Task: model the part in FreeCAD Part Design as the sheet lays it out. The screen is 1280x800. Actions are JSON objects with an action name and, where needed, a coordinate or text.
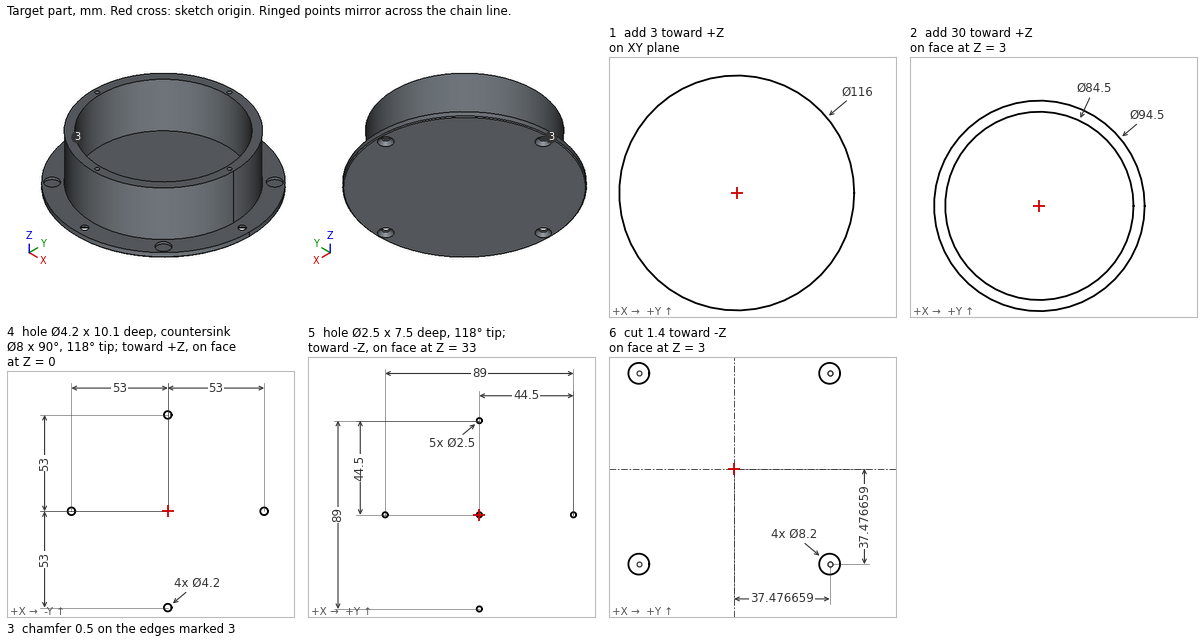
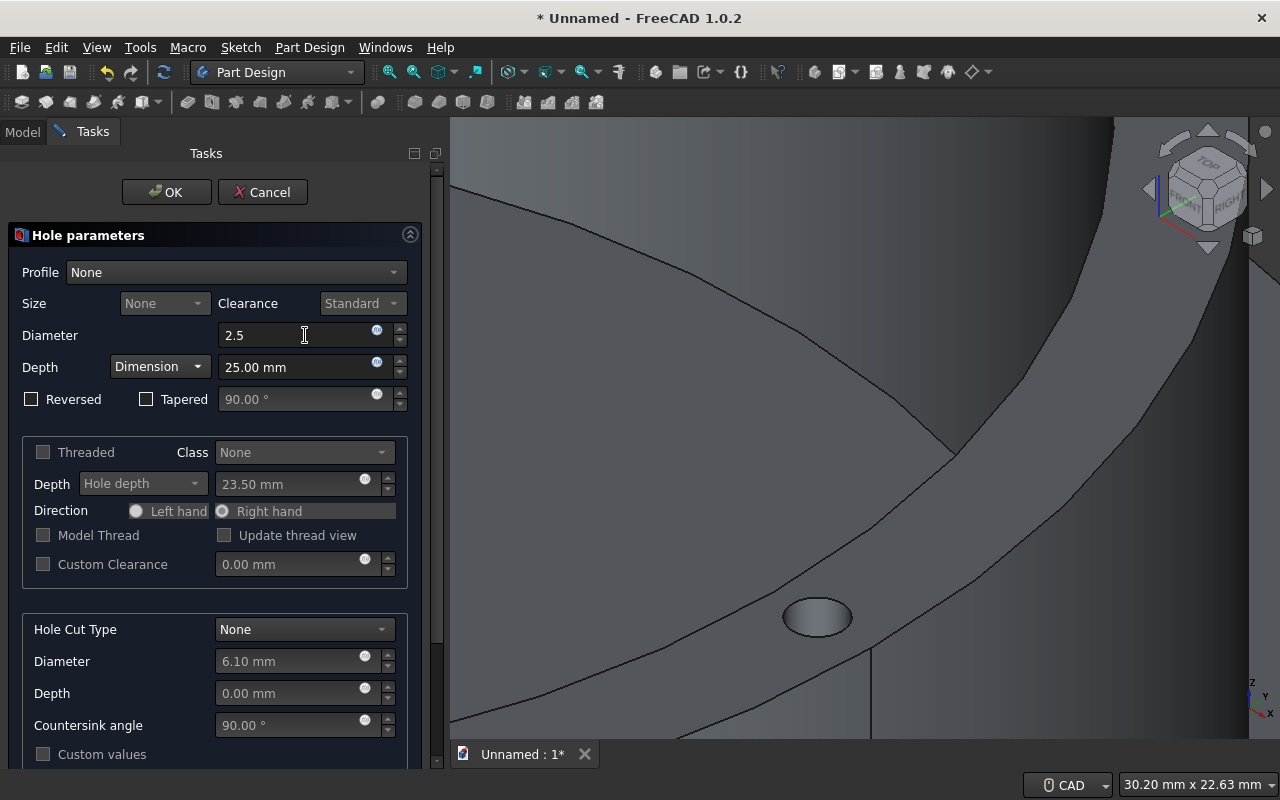
{"action": "triple_click", "coordinate": [305, 367]}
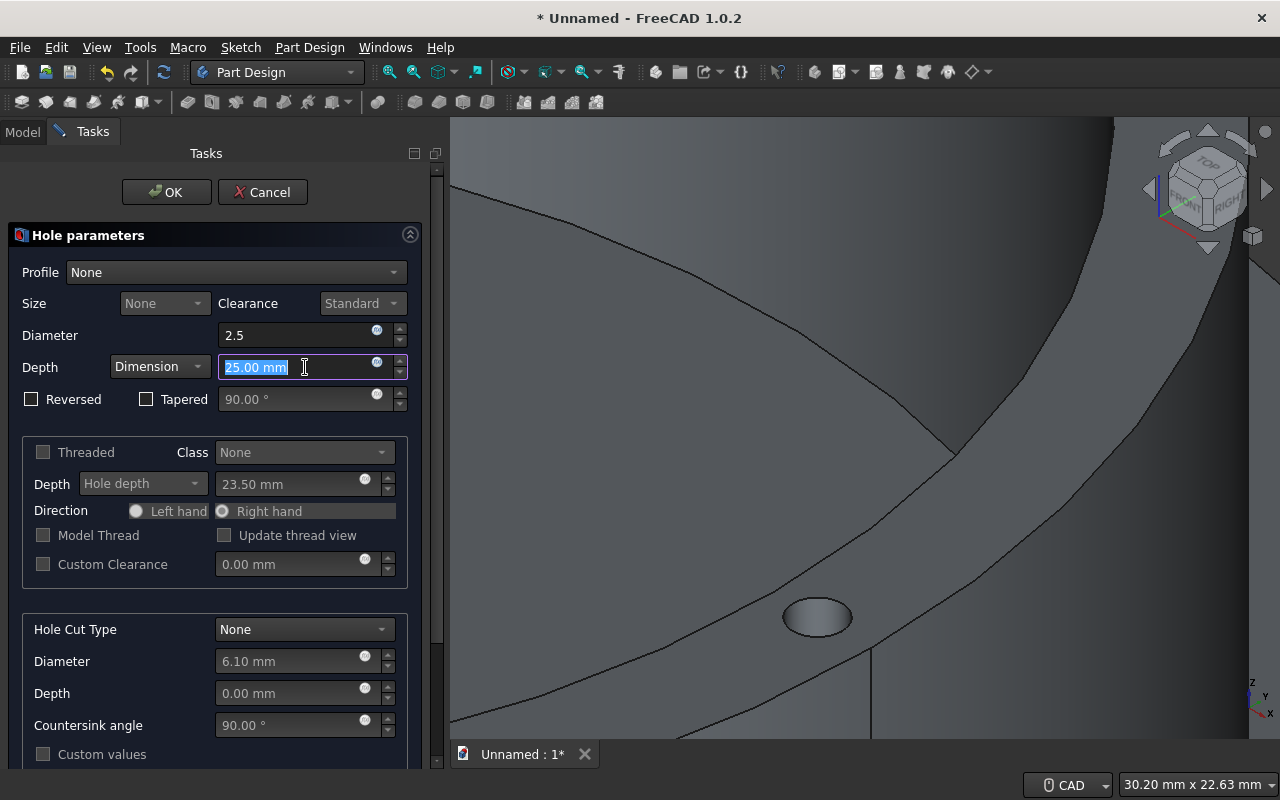
{"action": "type", "text": "7.5"}
{"action": "key", "text": "Tab"}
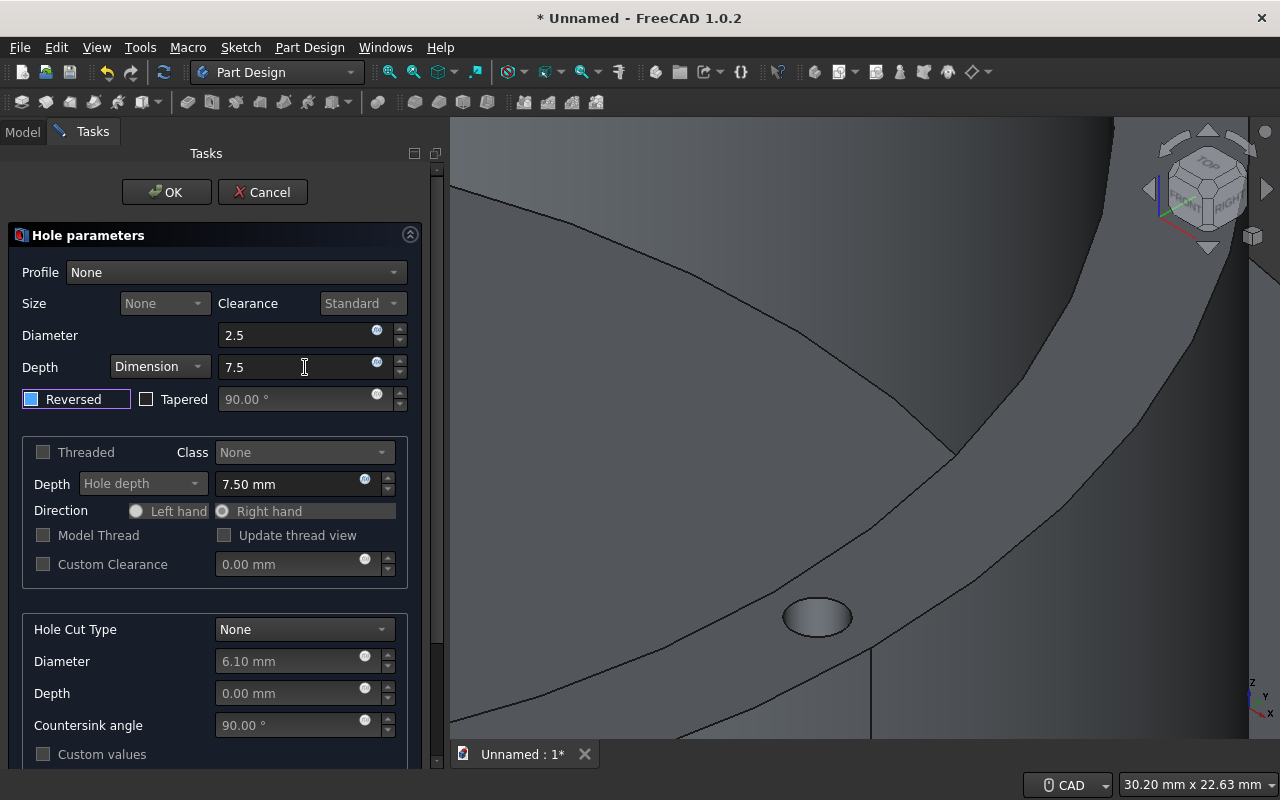
{"action": "left_click", "coordinate": [167, 192]}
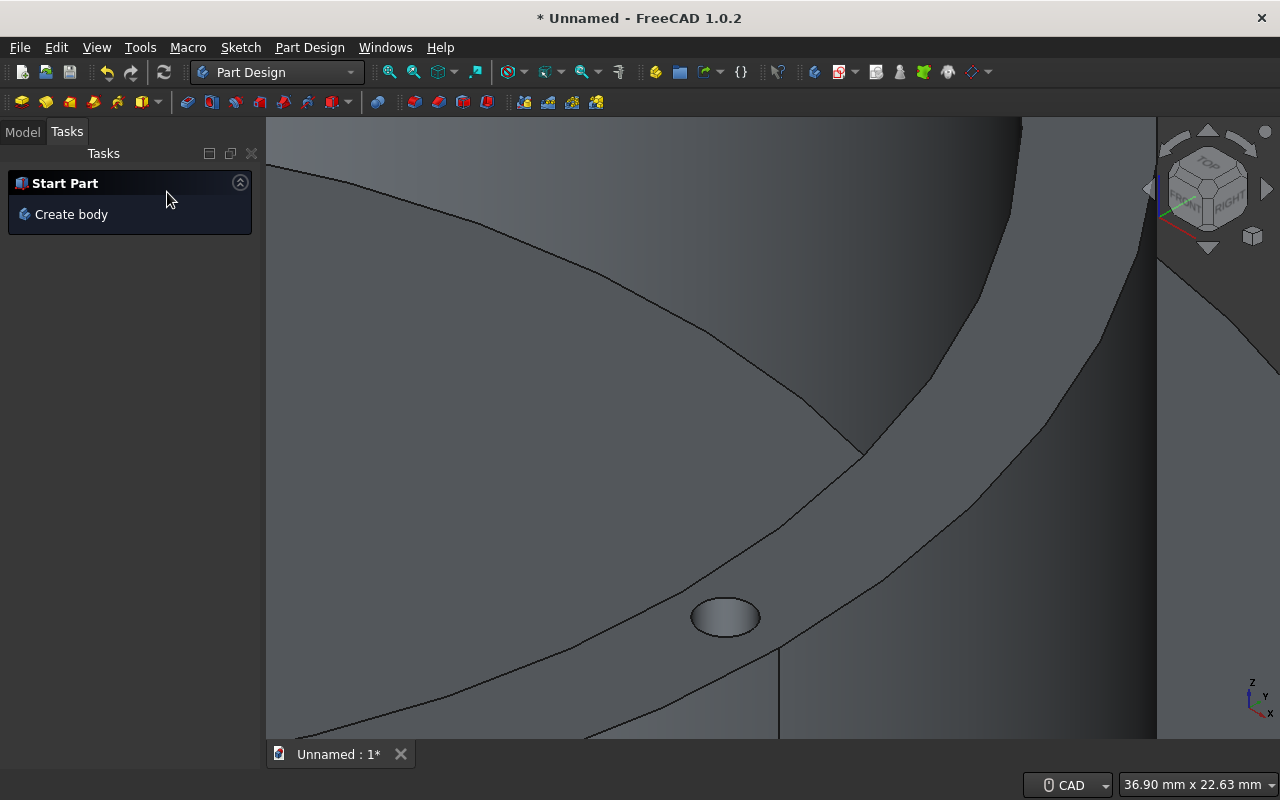
{"action": "left_click", "coordinate": [390, 72]}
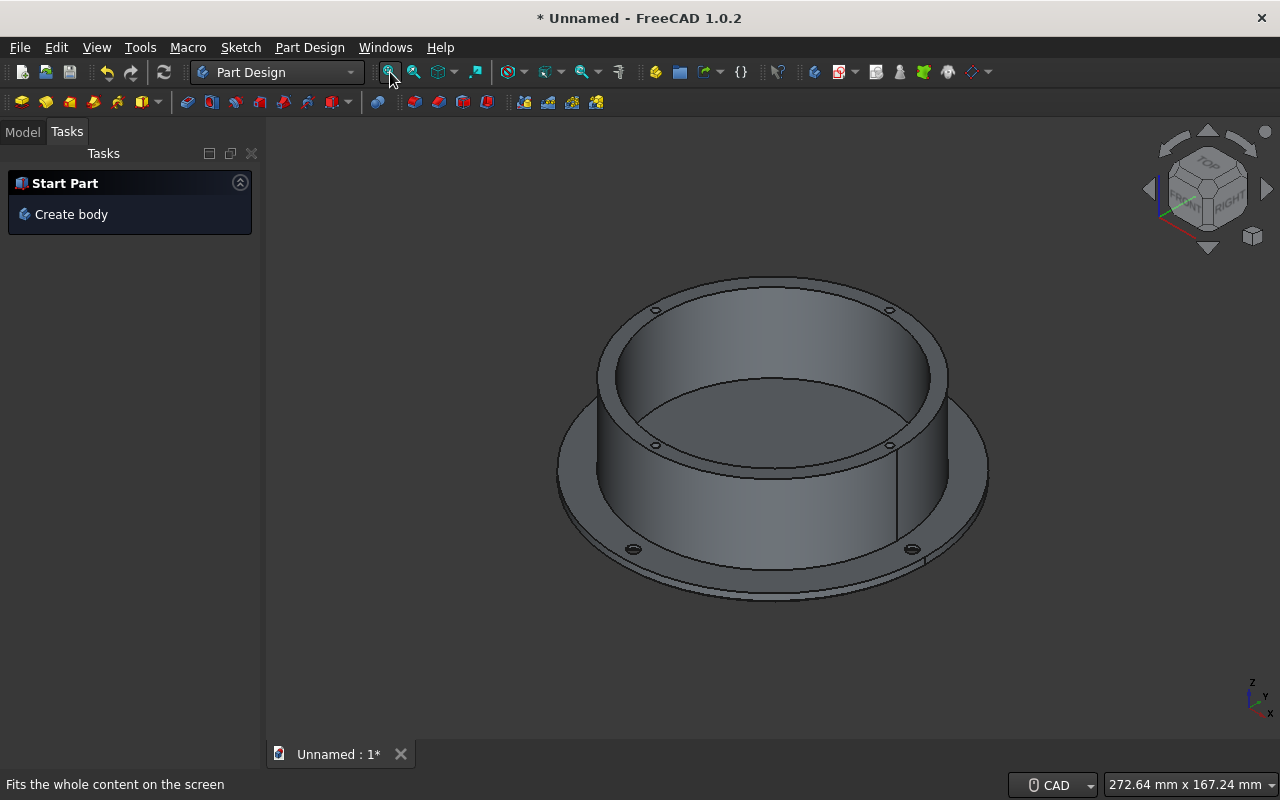
{"action": "left_click", "coordinate": [805, 450]}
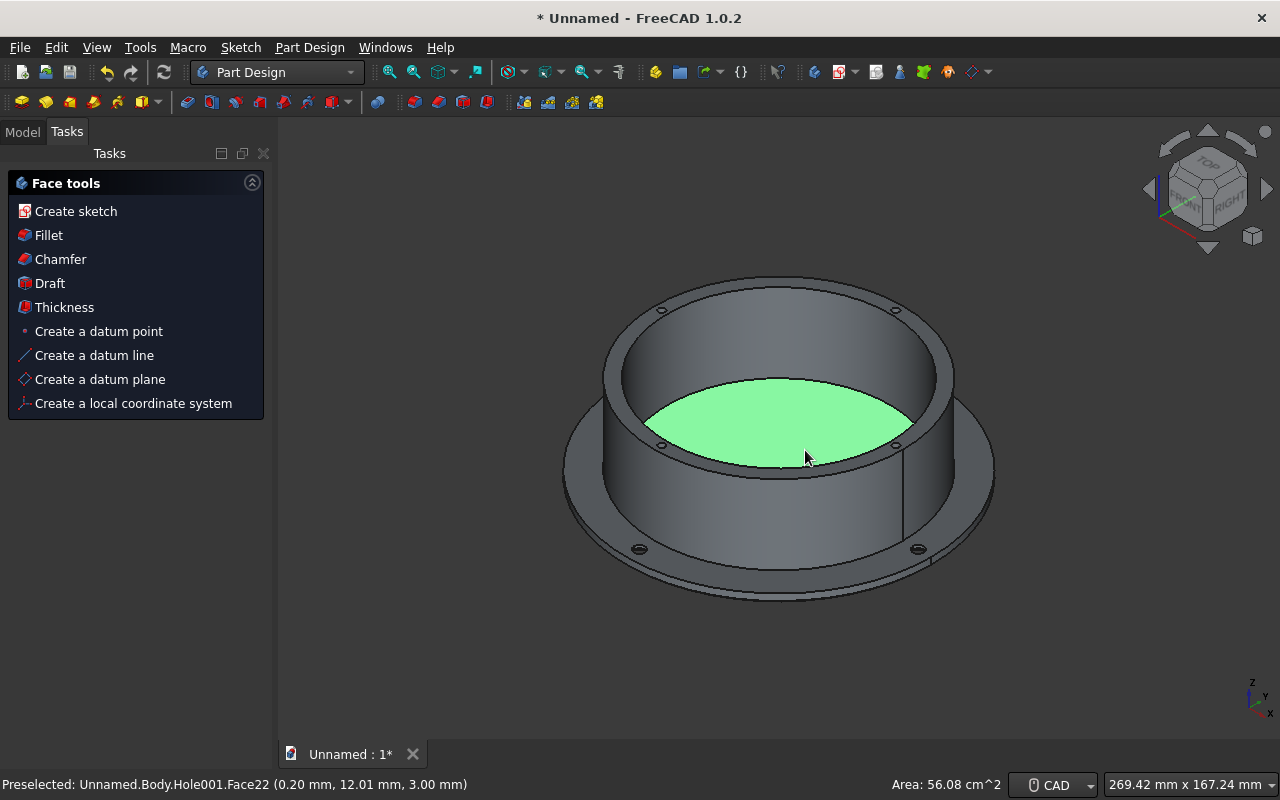
{"action": "left_click", "coordinate": [840, 72]}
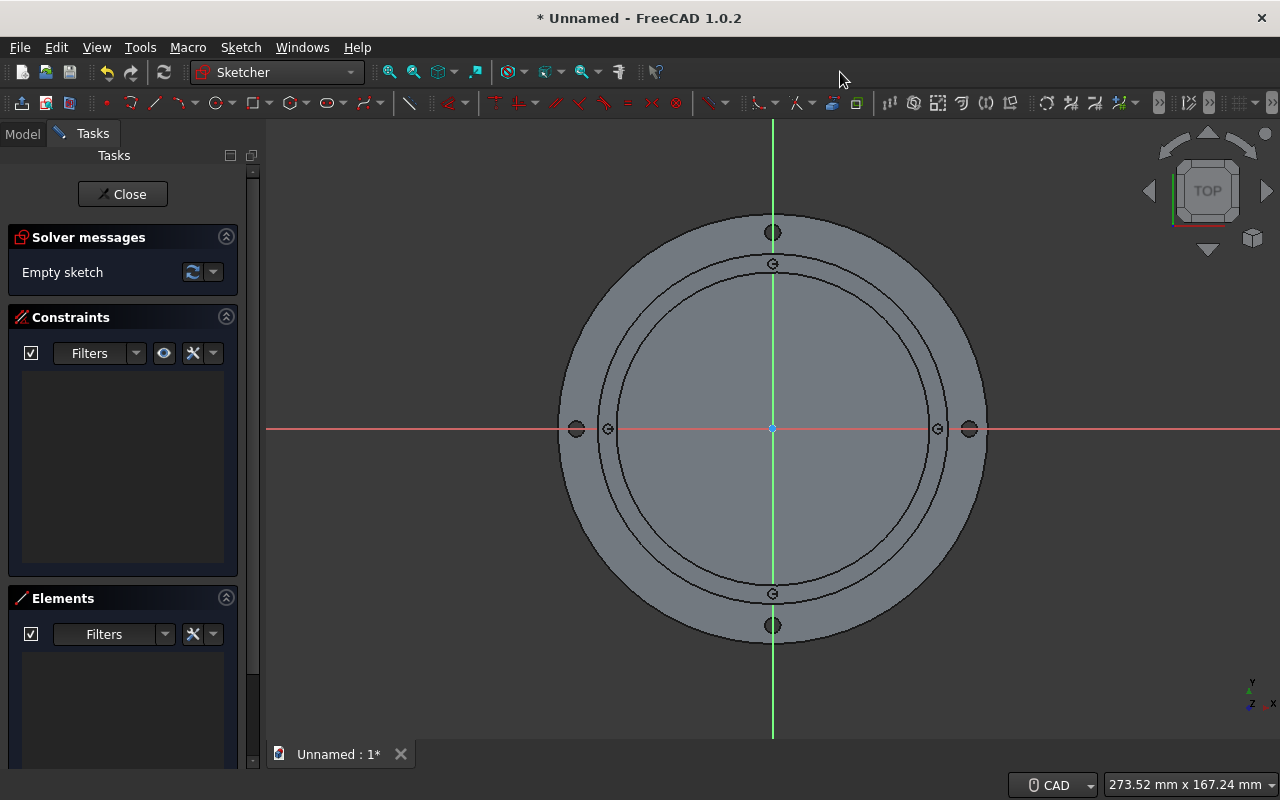
{"action": "left_click", "coordinate": [216, 104]}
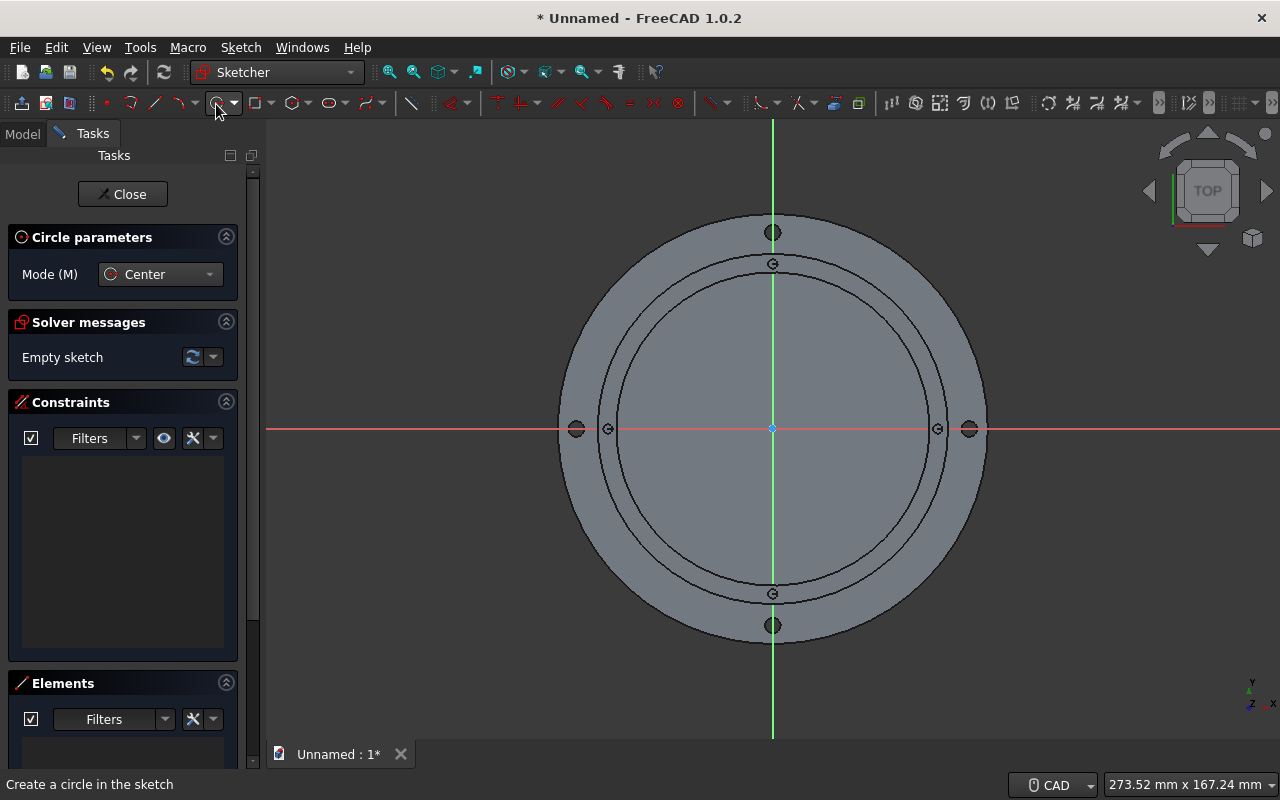
{"action": "scroll", "coordinate": [912, 568], "scroll_direction": "up", "scroll_amount": 3}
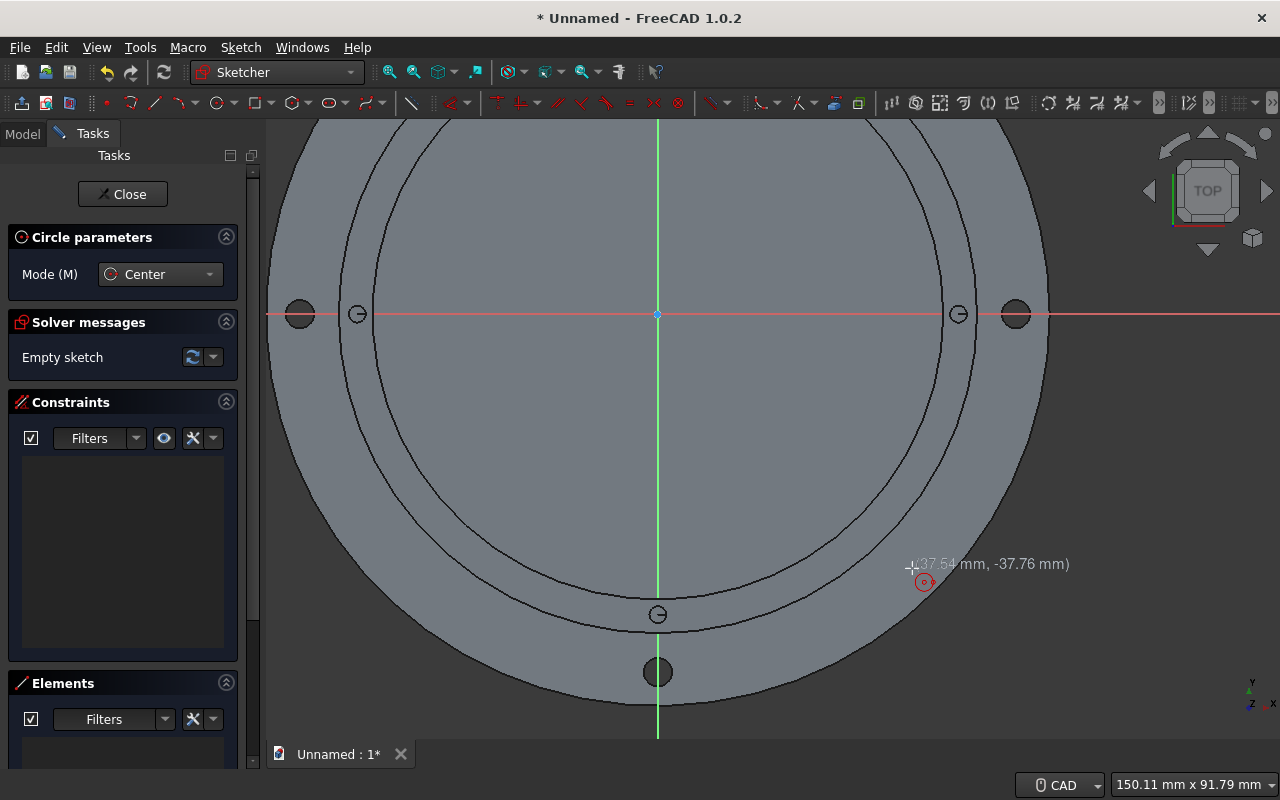
{"action": "left_click", "coordinate": [911, 567]}
{"action": "mouse_move", "coordinate": [931, 548]}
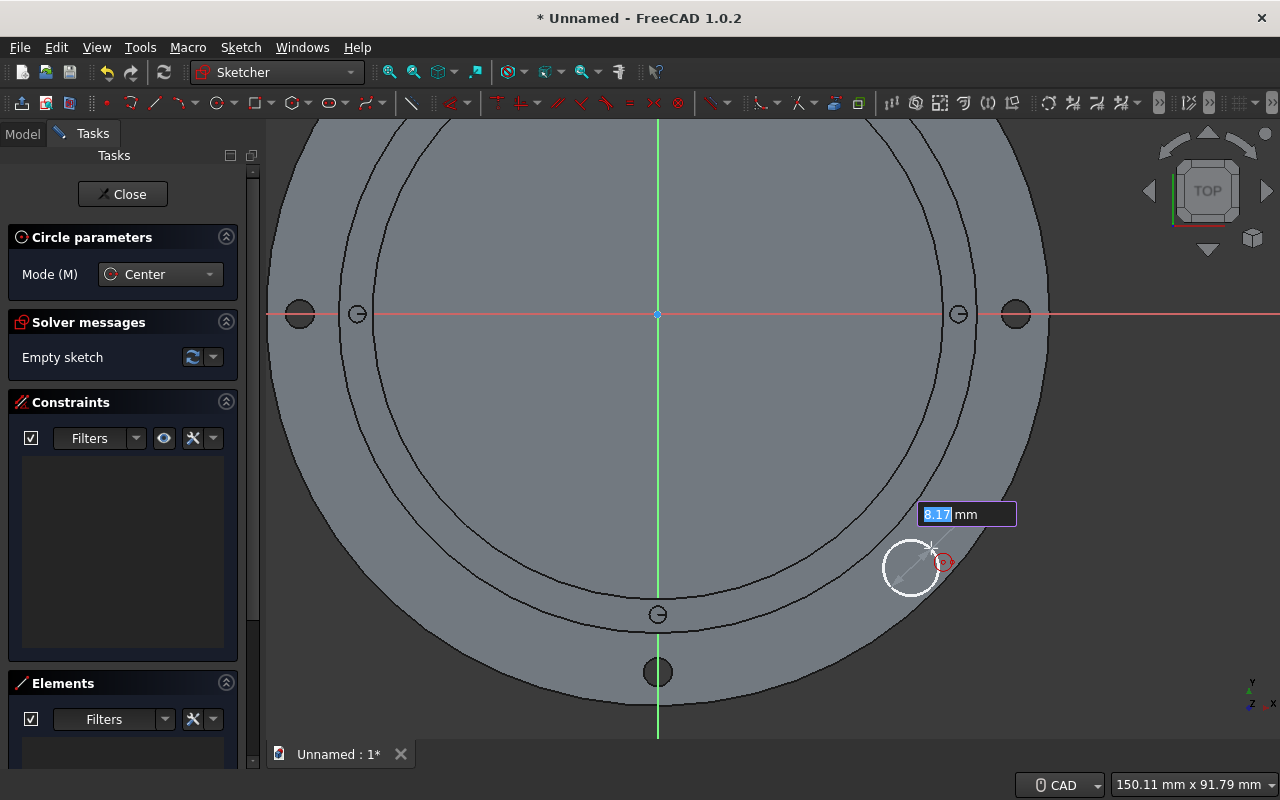
{"action": "type", "text": "8.2"}
{"action": "key", "text": "Return"}